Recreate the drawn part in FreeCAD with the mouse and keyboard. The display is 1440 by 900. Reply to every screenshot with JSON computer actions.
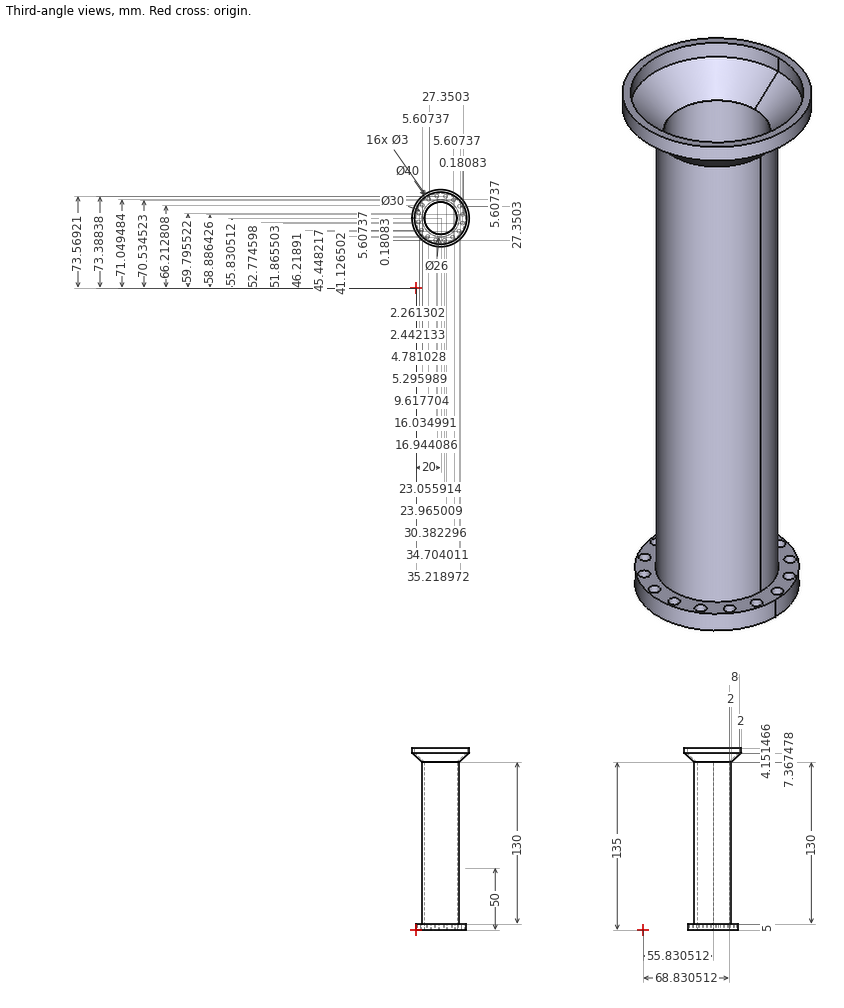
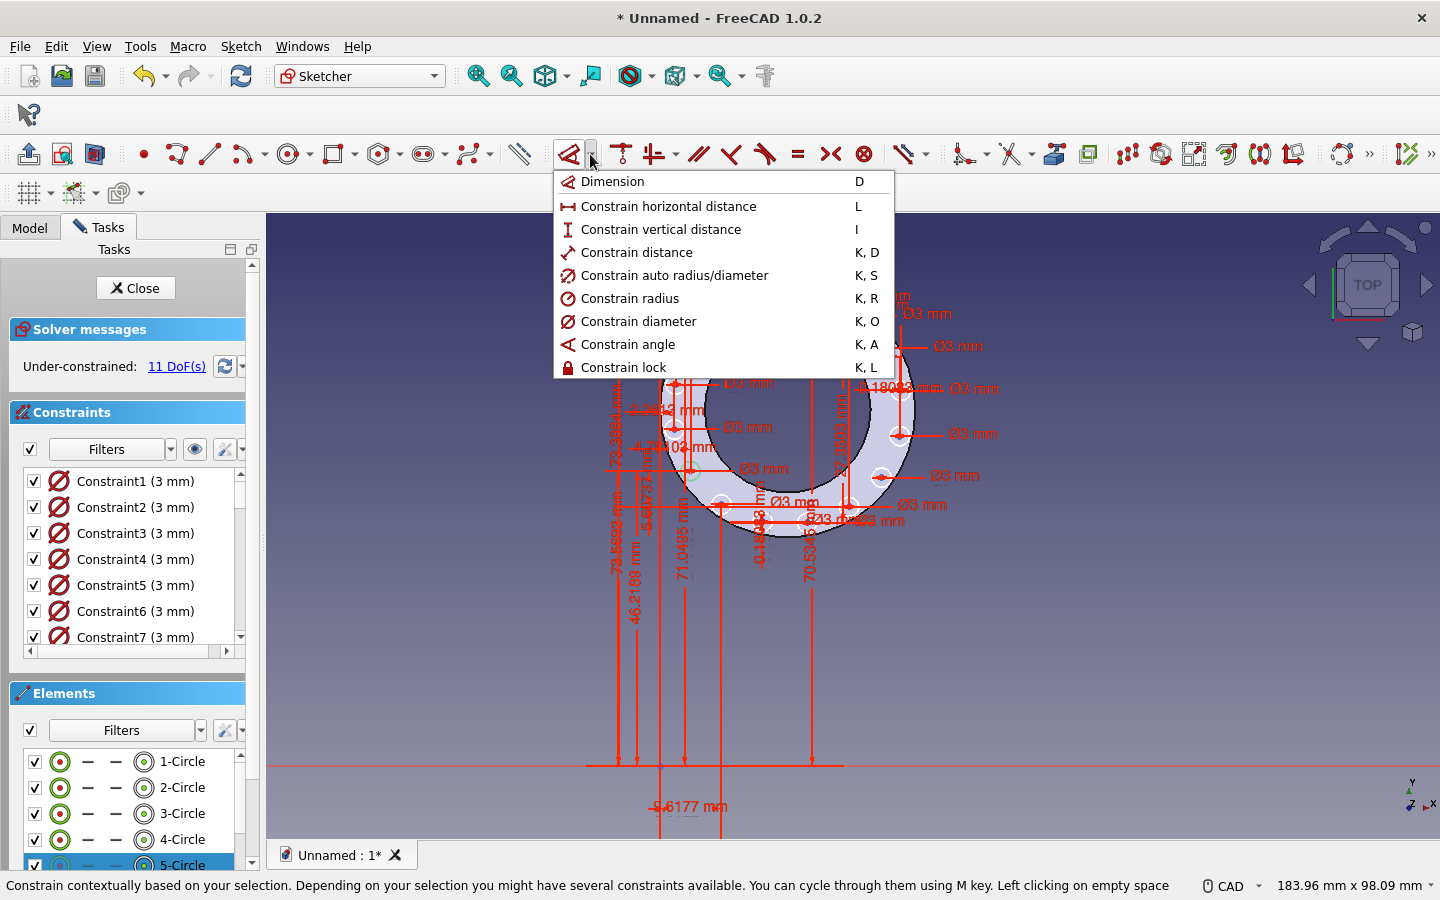
{"action": "left_click", "coordinate": [724, 206]}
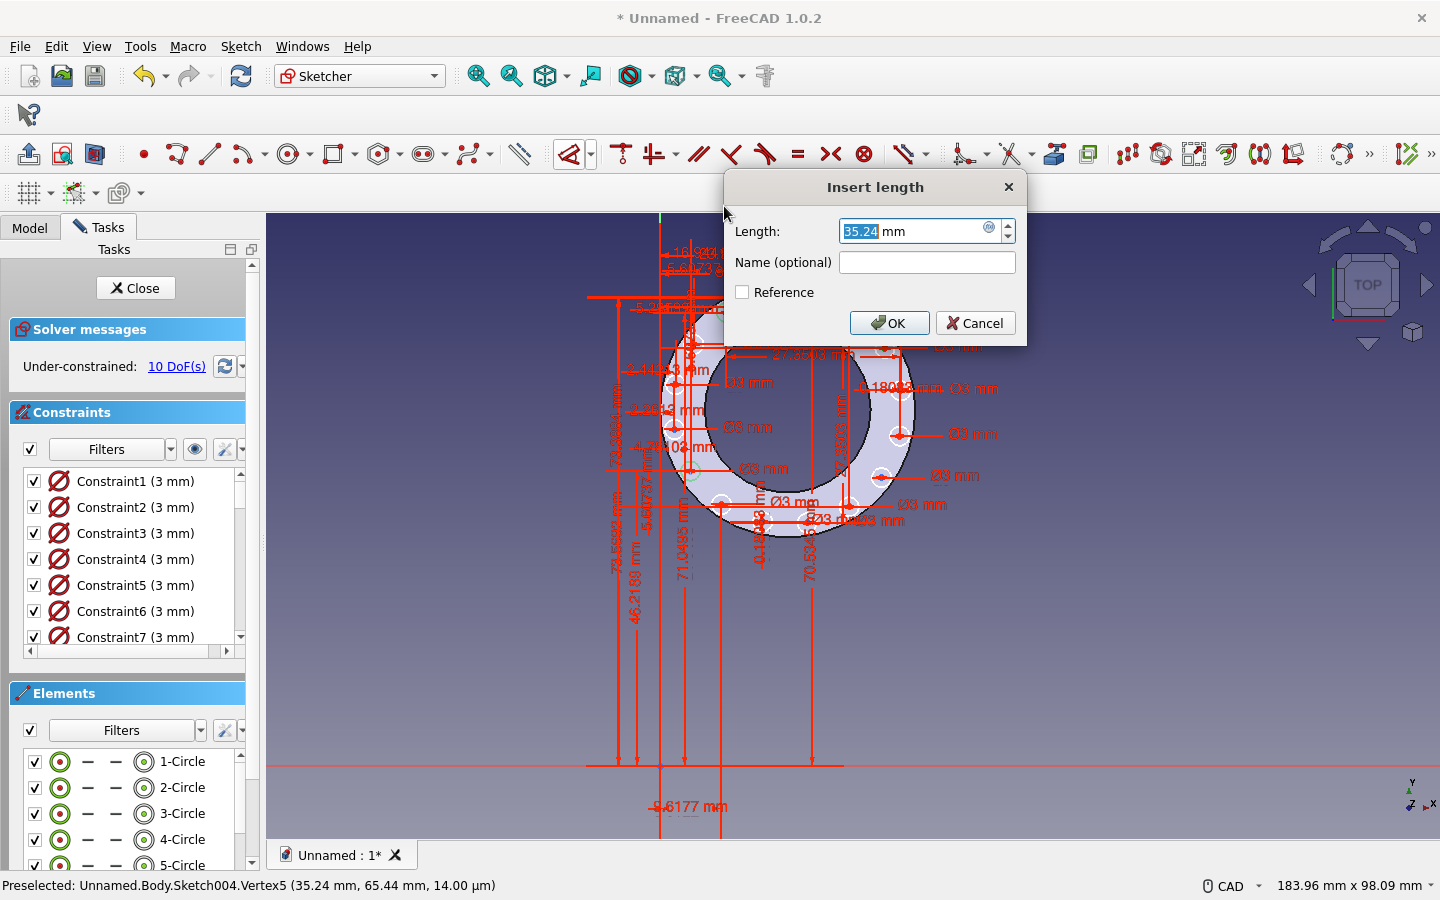
{"action": "type", "text": "35.218972"}
{"action": "key", "text": "Return"}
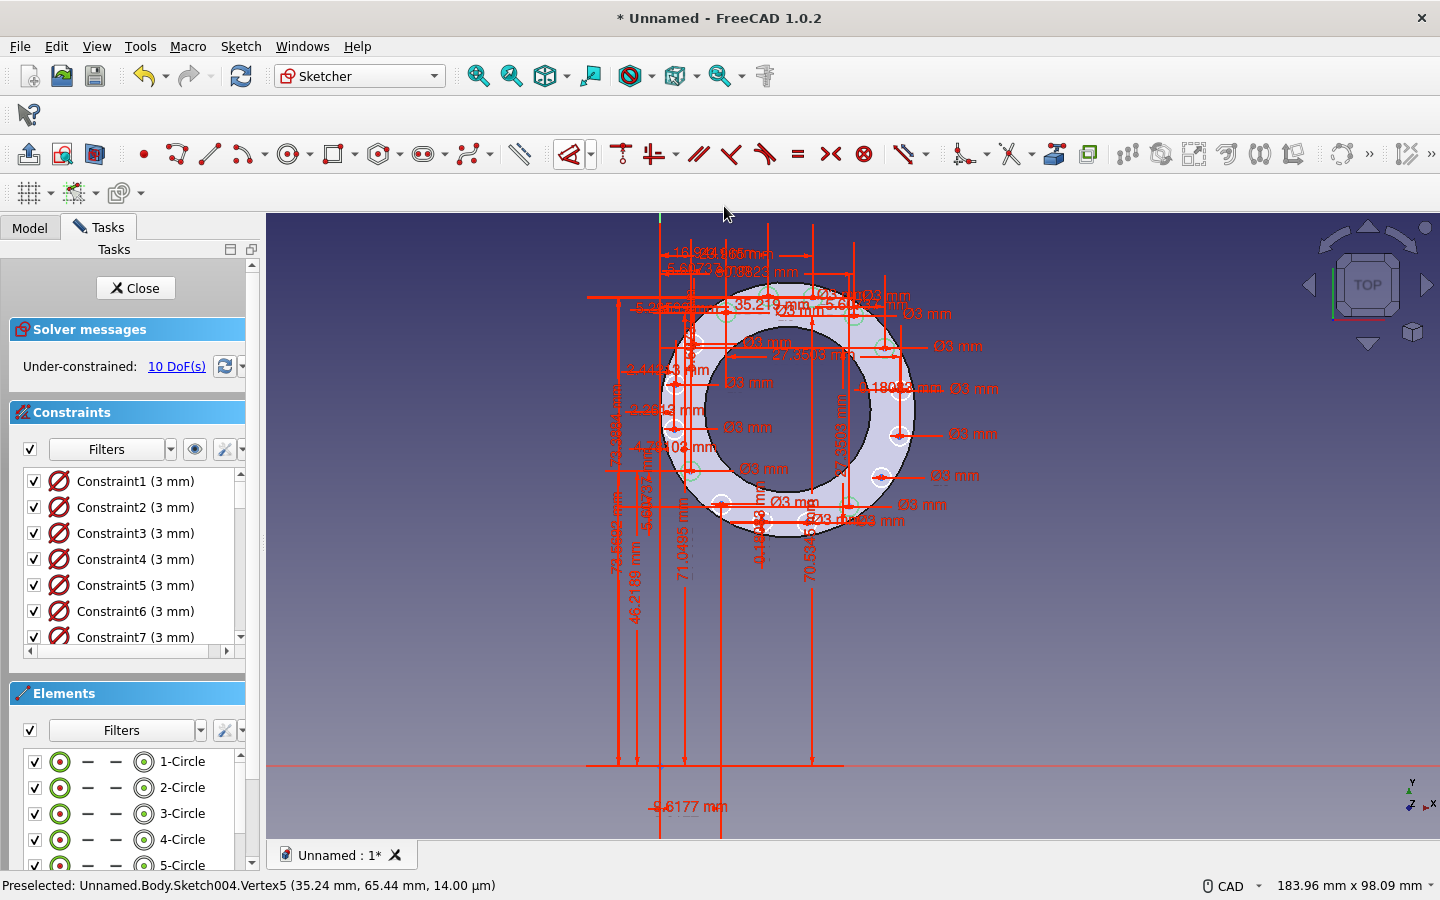
{"action": "left_click", "coordinate": [901, 391]}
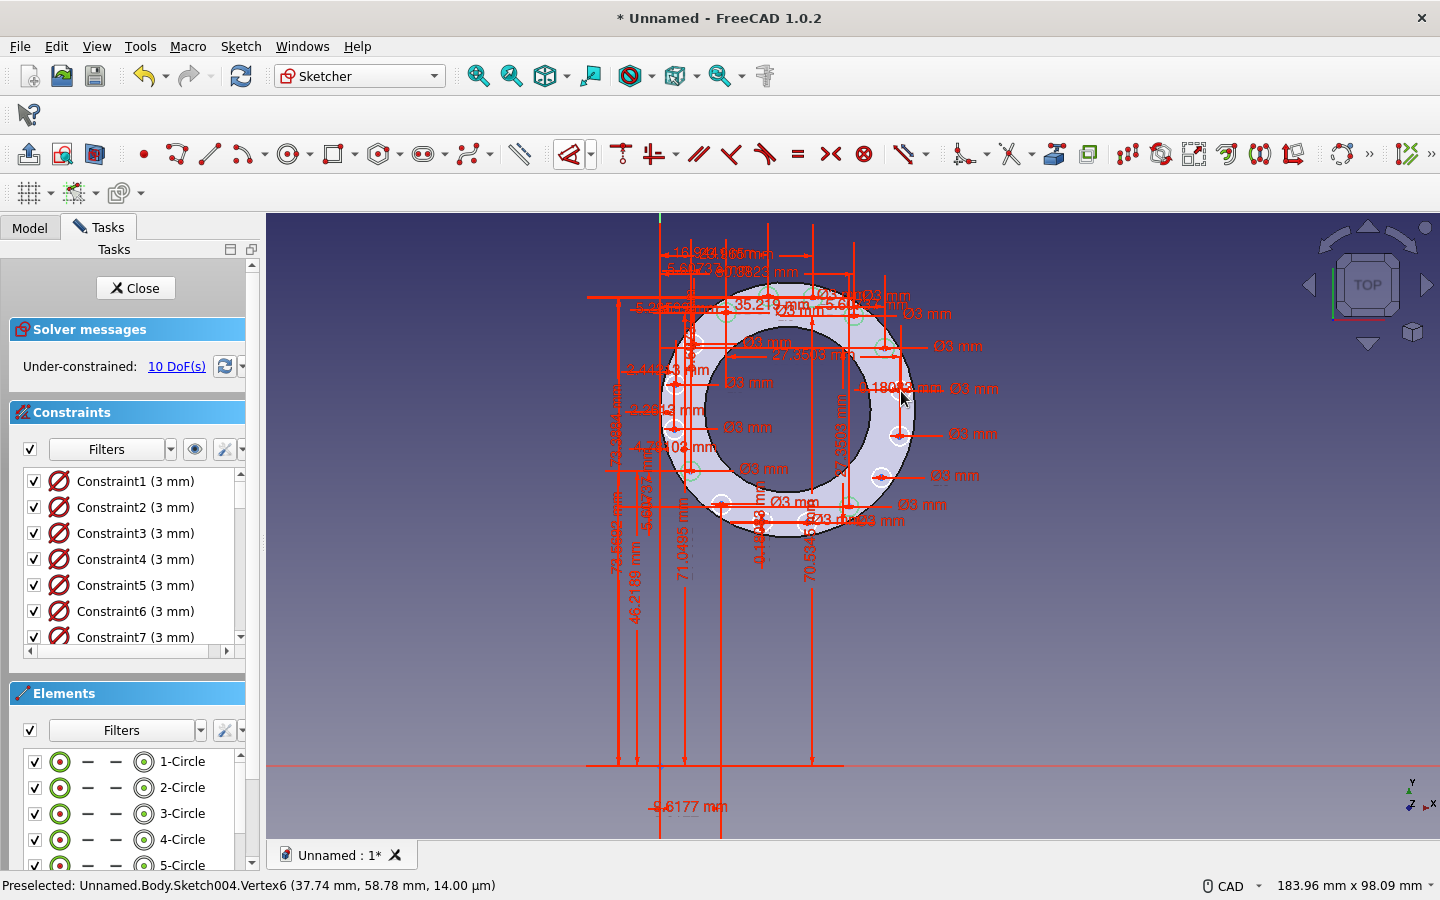
{"action": "key", "text": "i"}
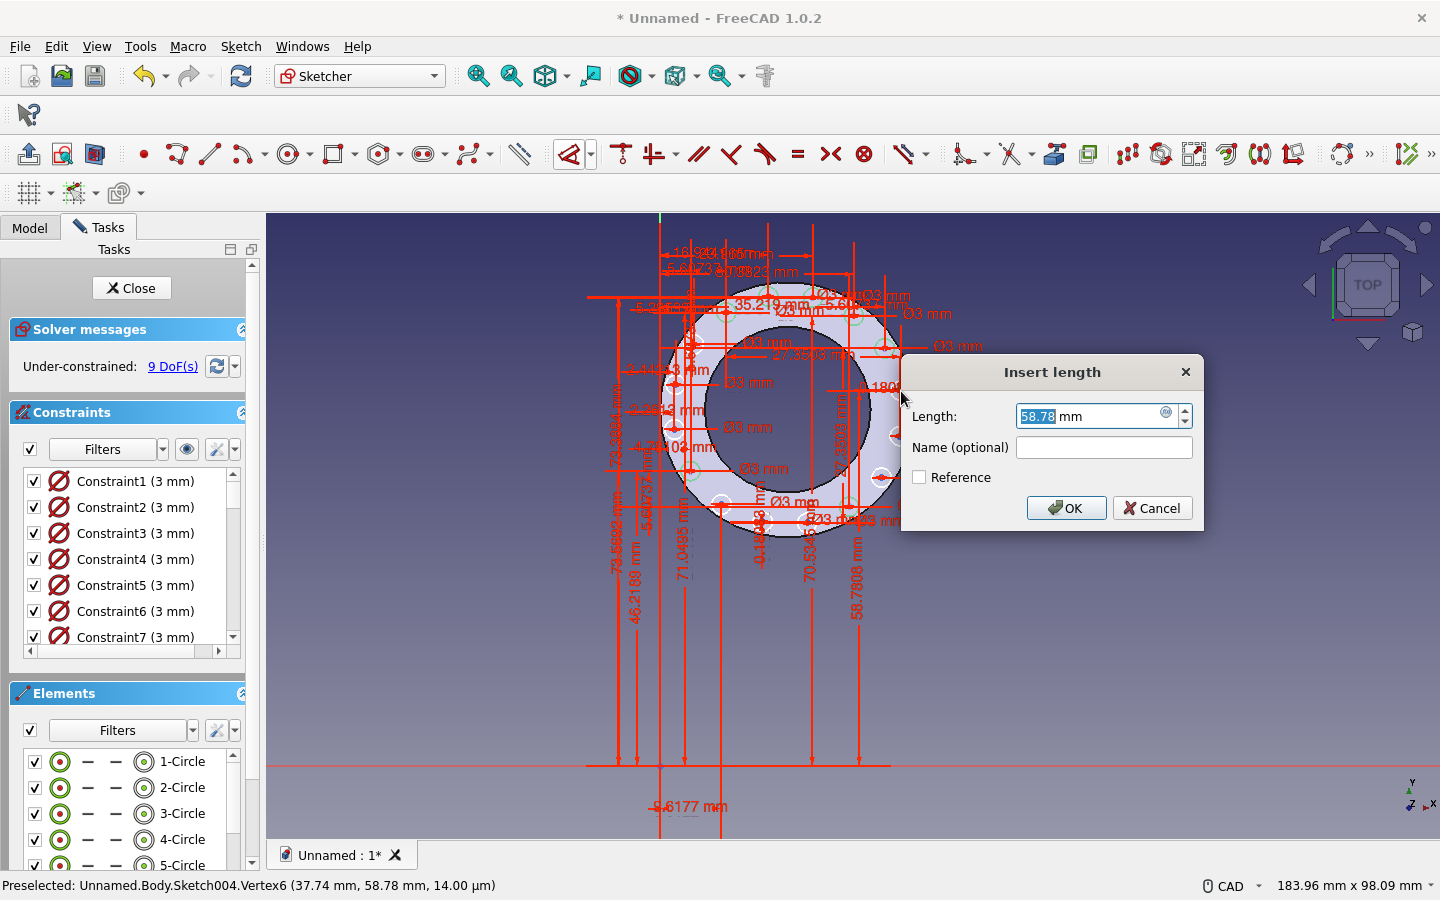
{"action": "type", "text": "58.886426"}
{"action": "key", "text": "Return"}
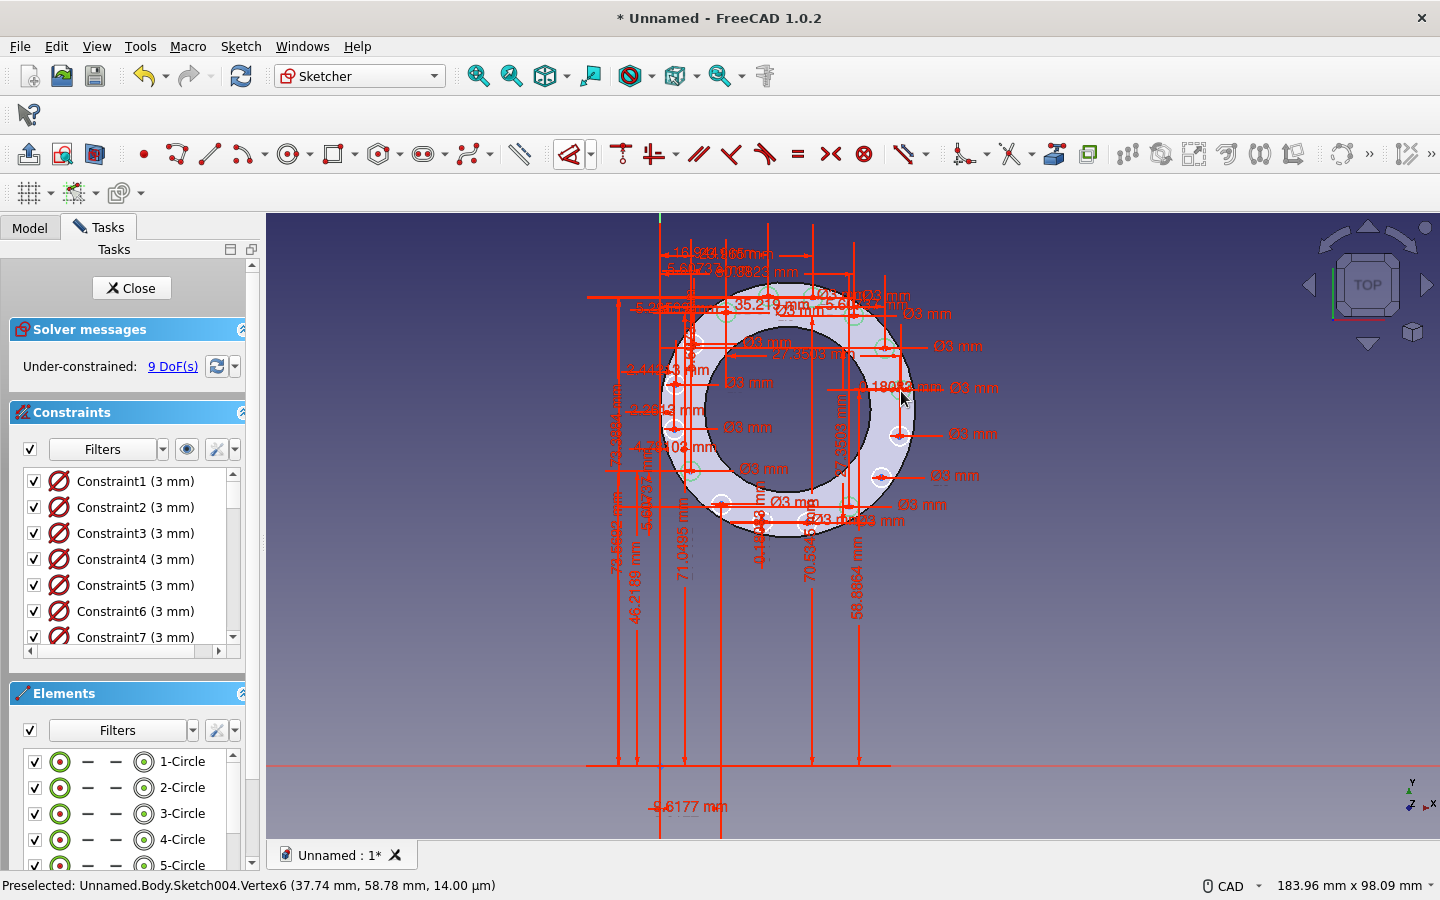
{"action": "left_click", "coordinate": [900, 436]}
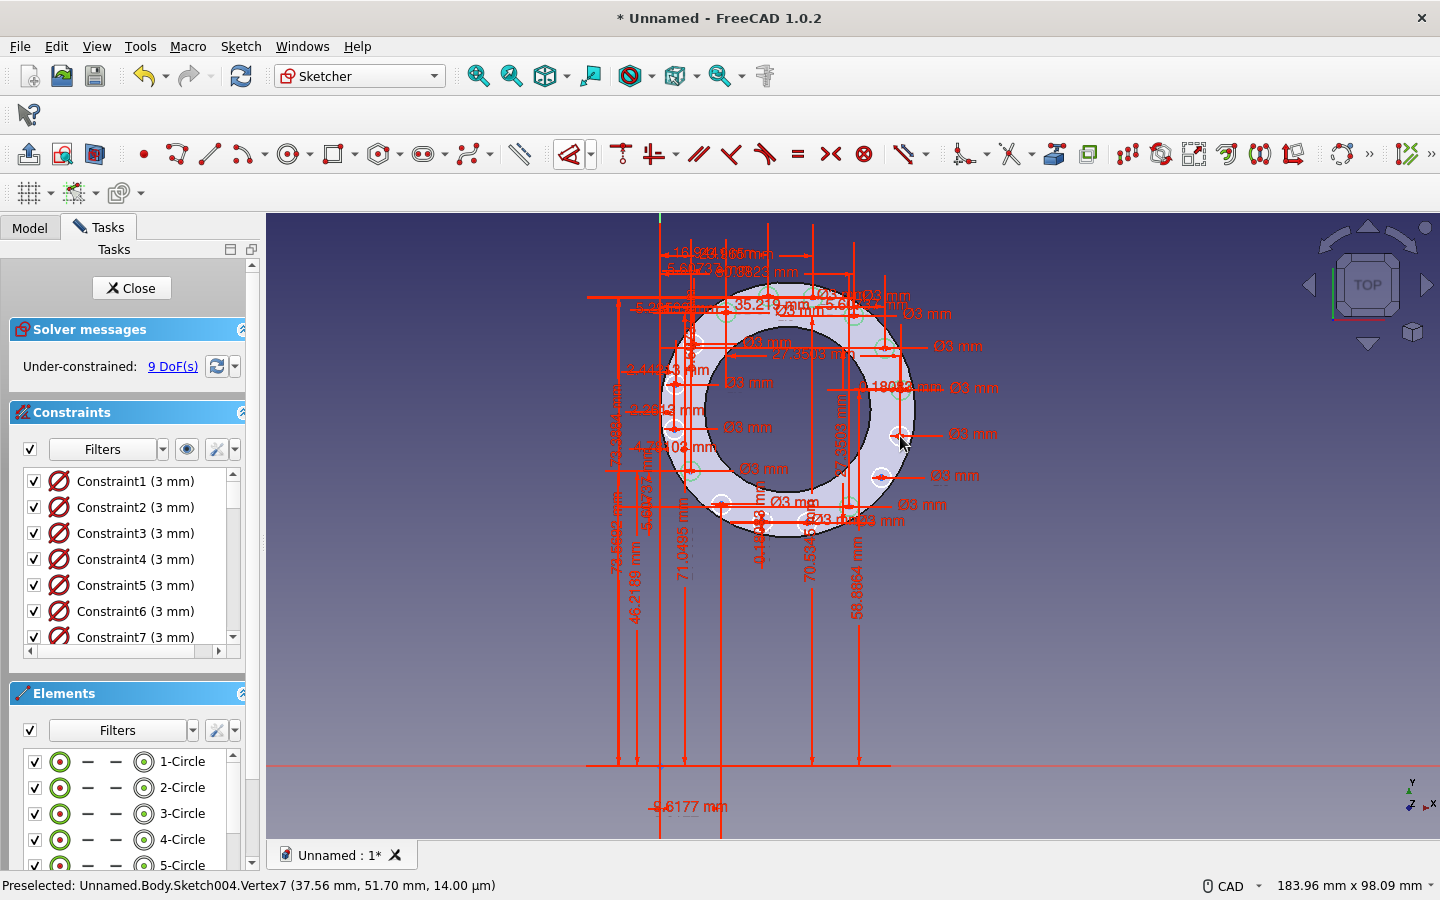
{"action": "left_click", "coordinate": [590, 154]}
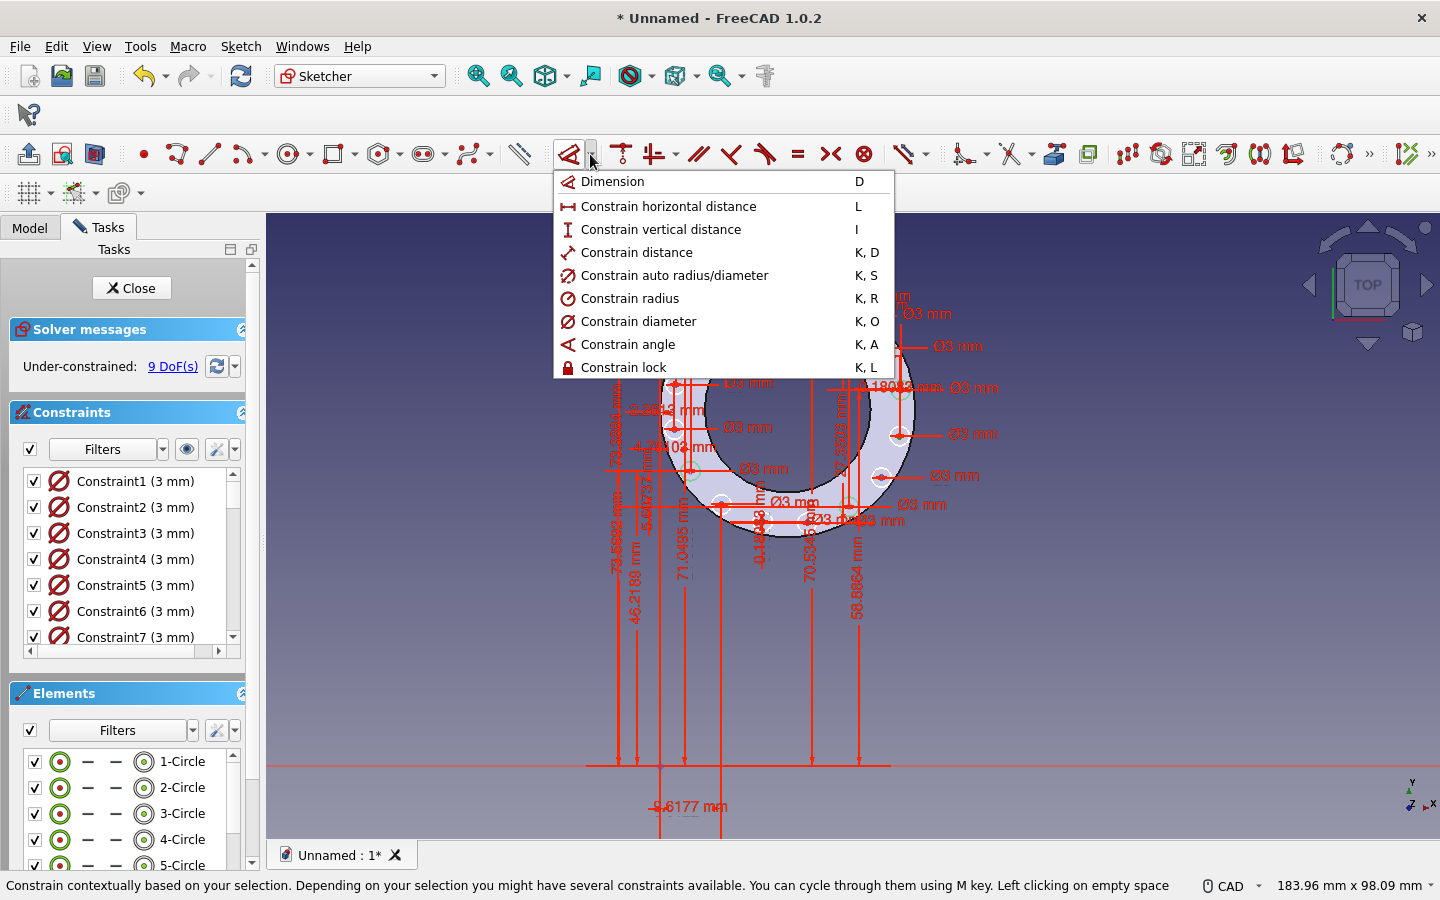
{"action": "left_click", "coordinate": [724, 230]}